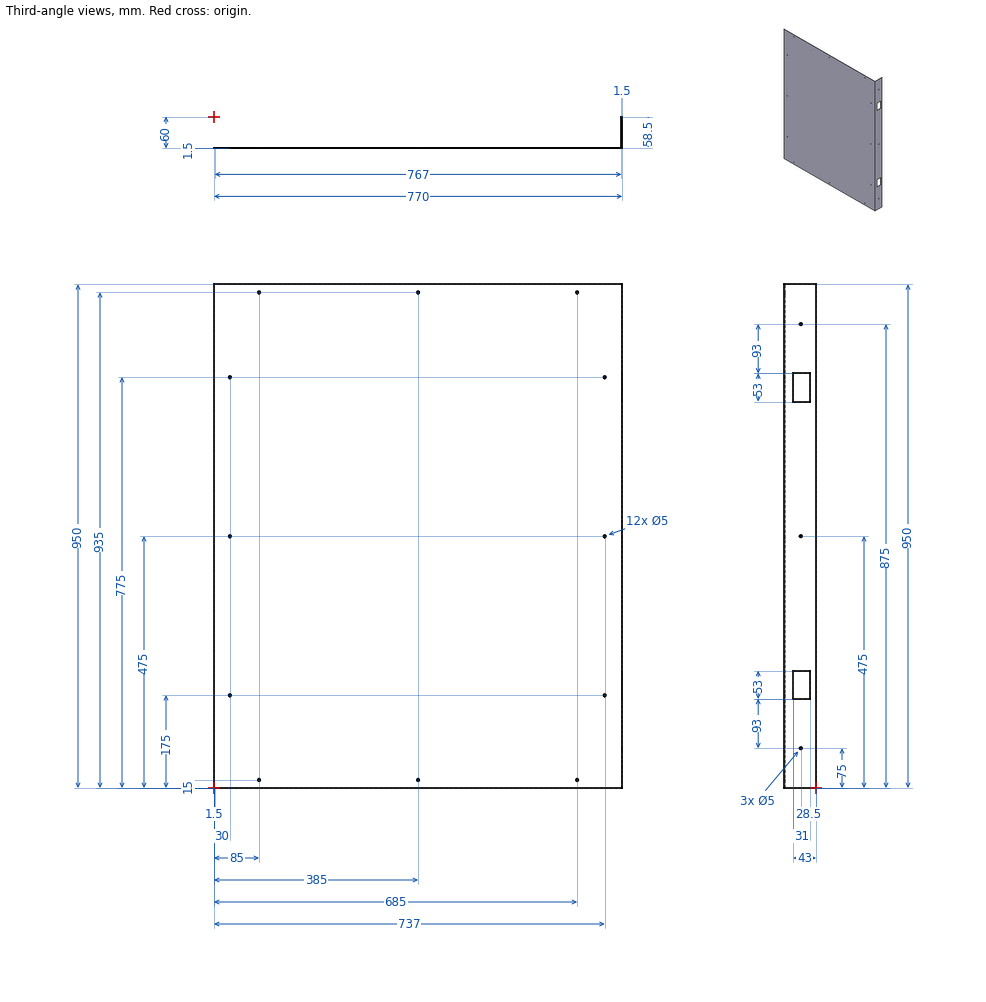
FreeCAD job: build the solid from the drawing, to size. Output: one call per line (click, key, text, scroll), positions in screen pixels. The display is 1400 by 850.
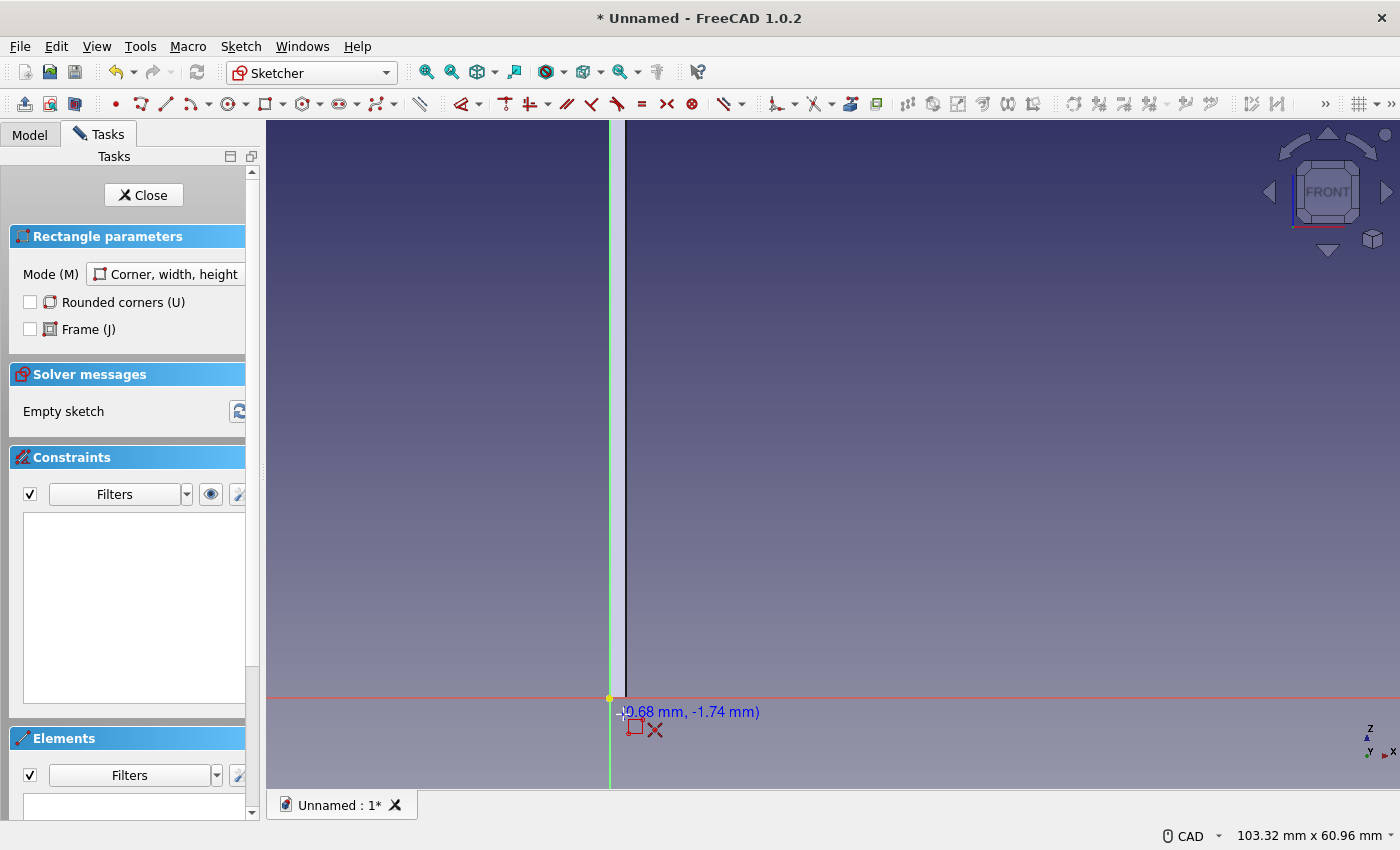
scroll(772, 715, down, 15)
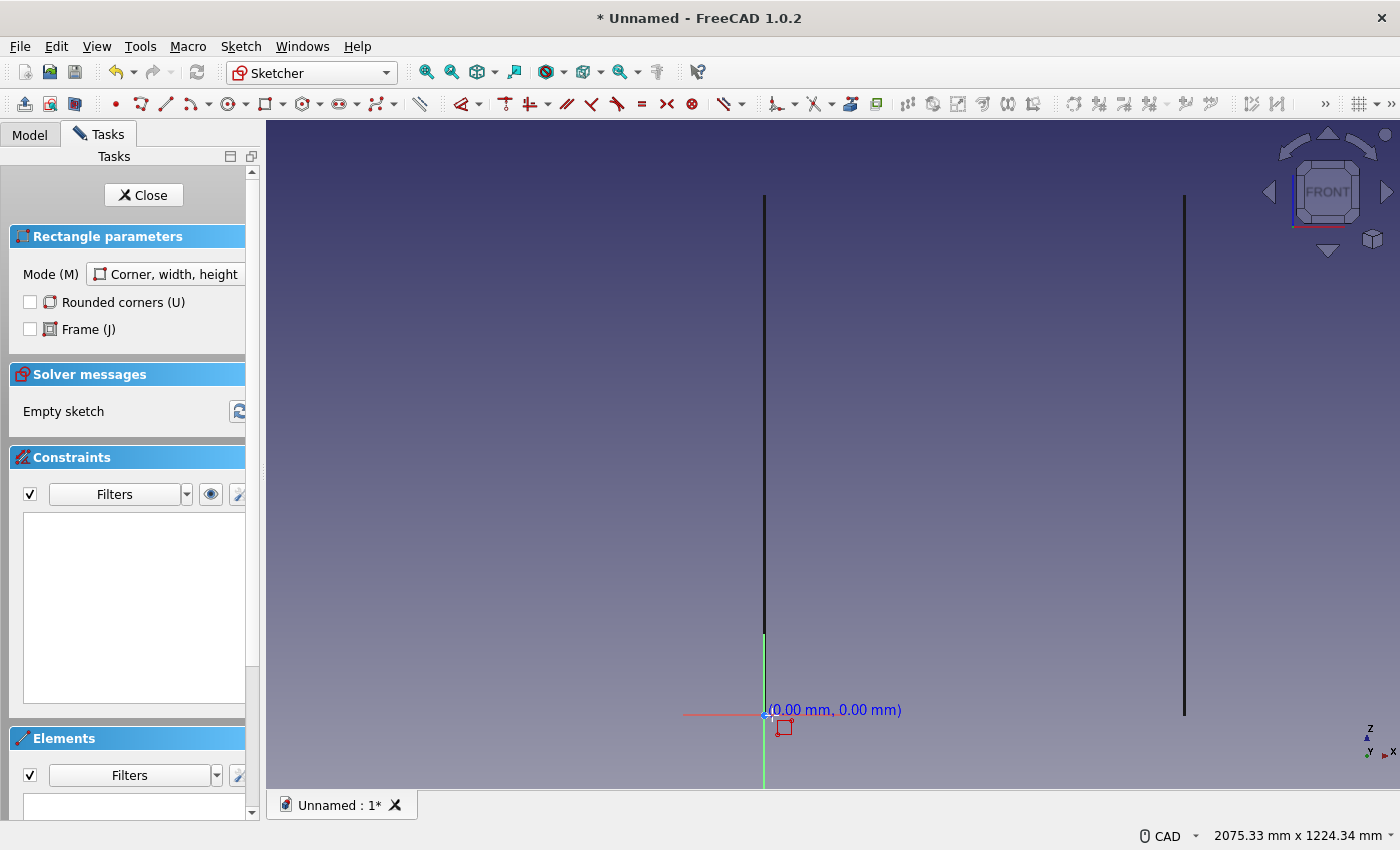
click(764, 715)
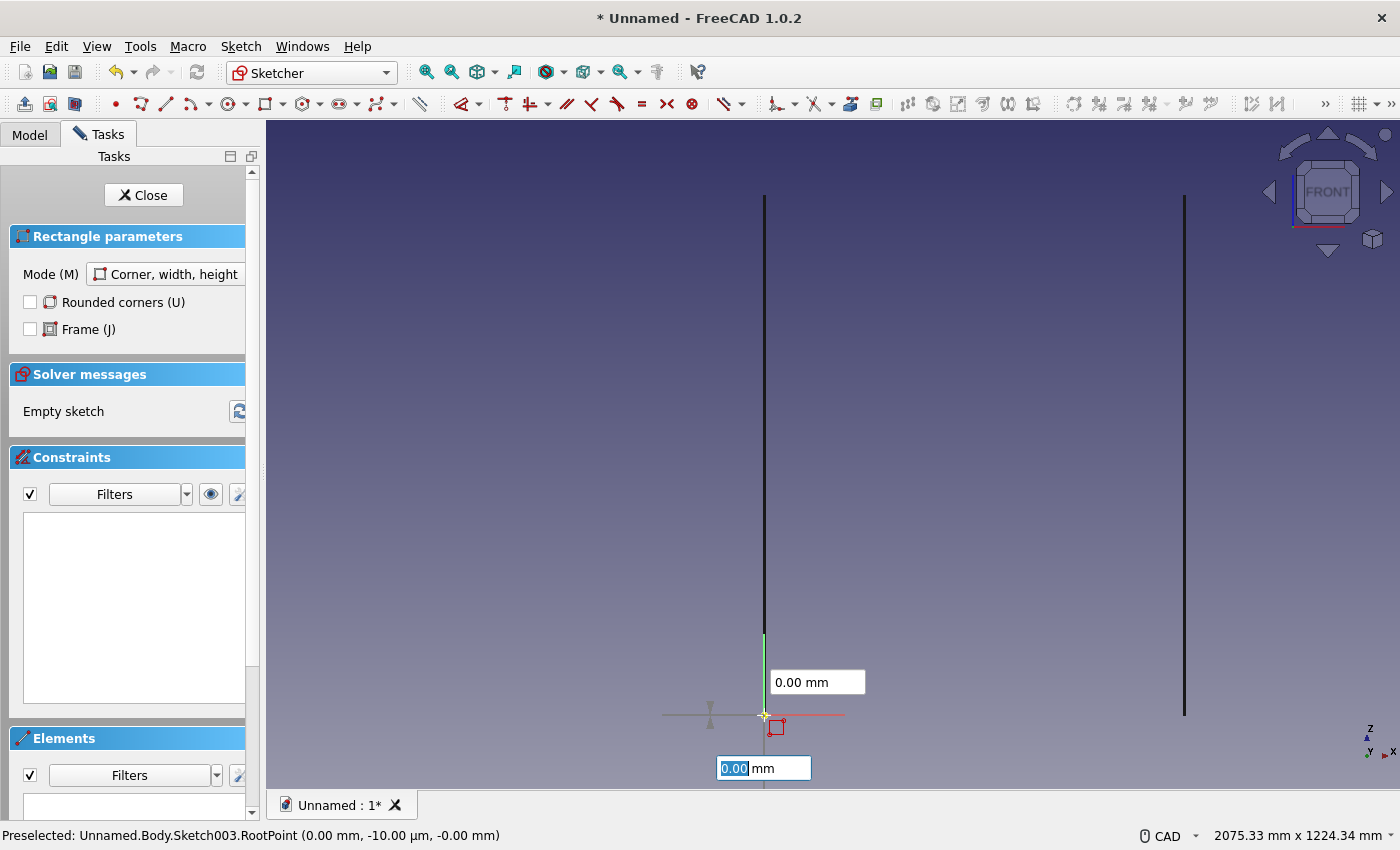
scroll(765, 196, up, 15)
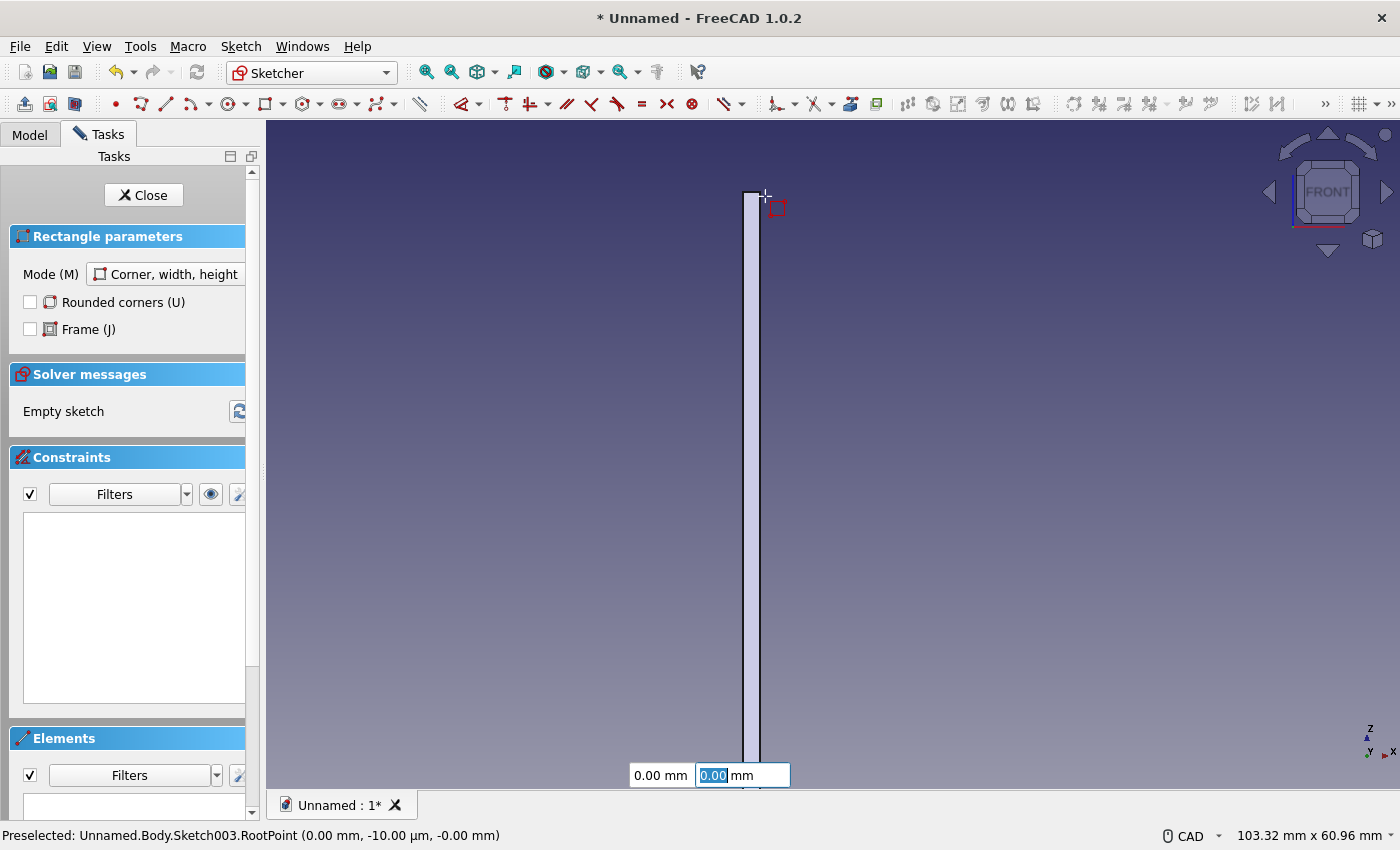
click(760, 192)
key(Escape)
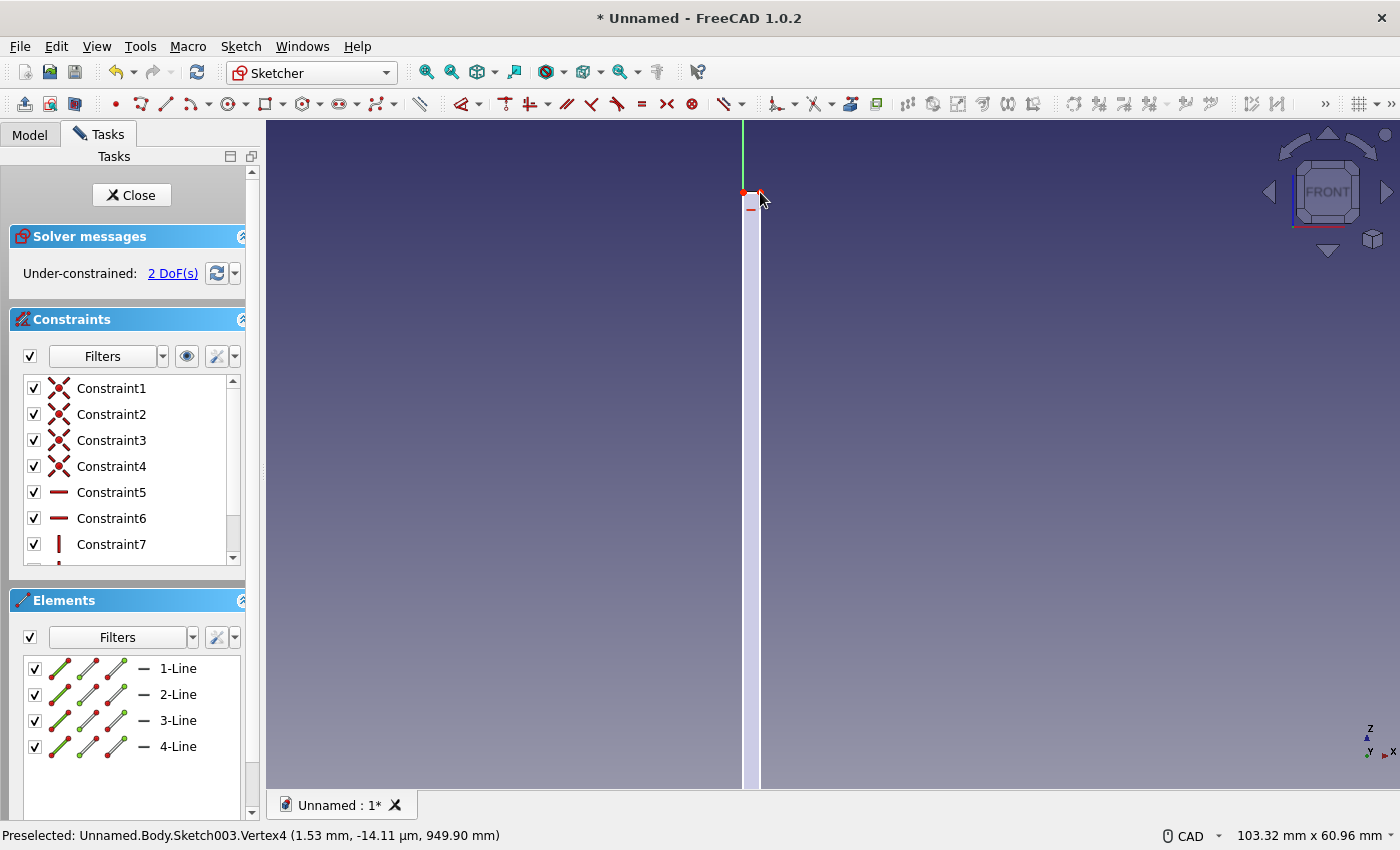
key(d)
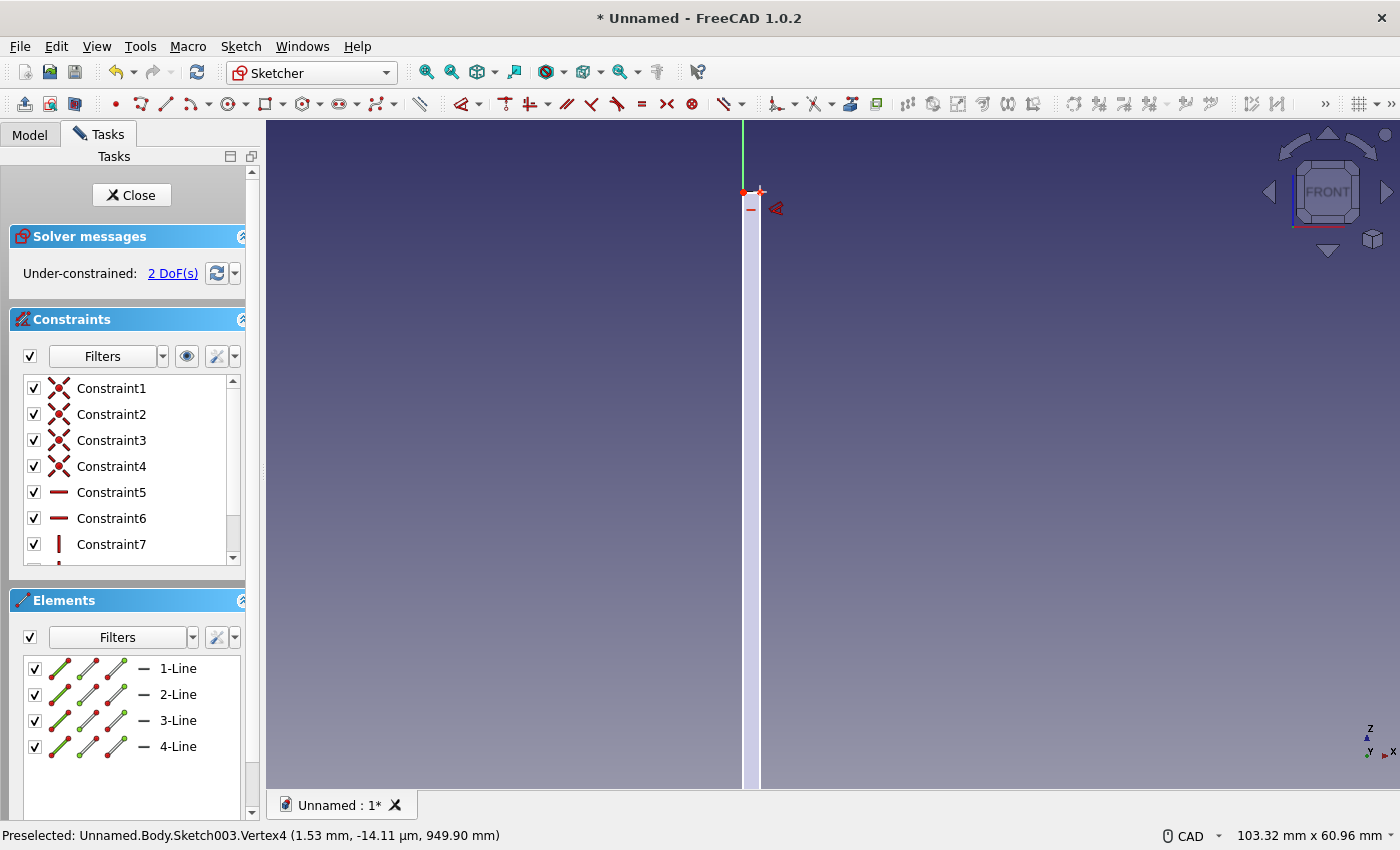
scroll(765, 195, down, 15)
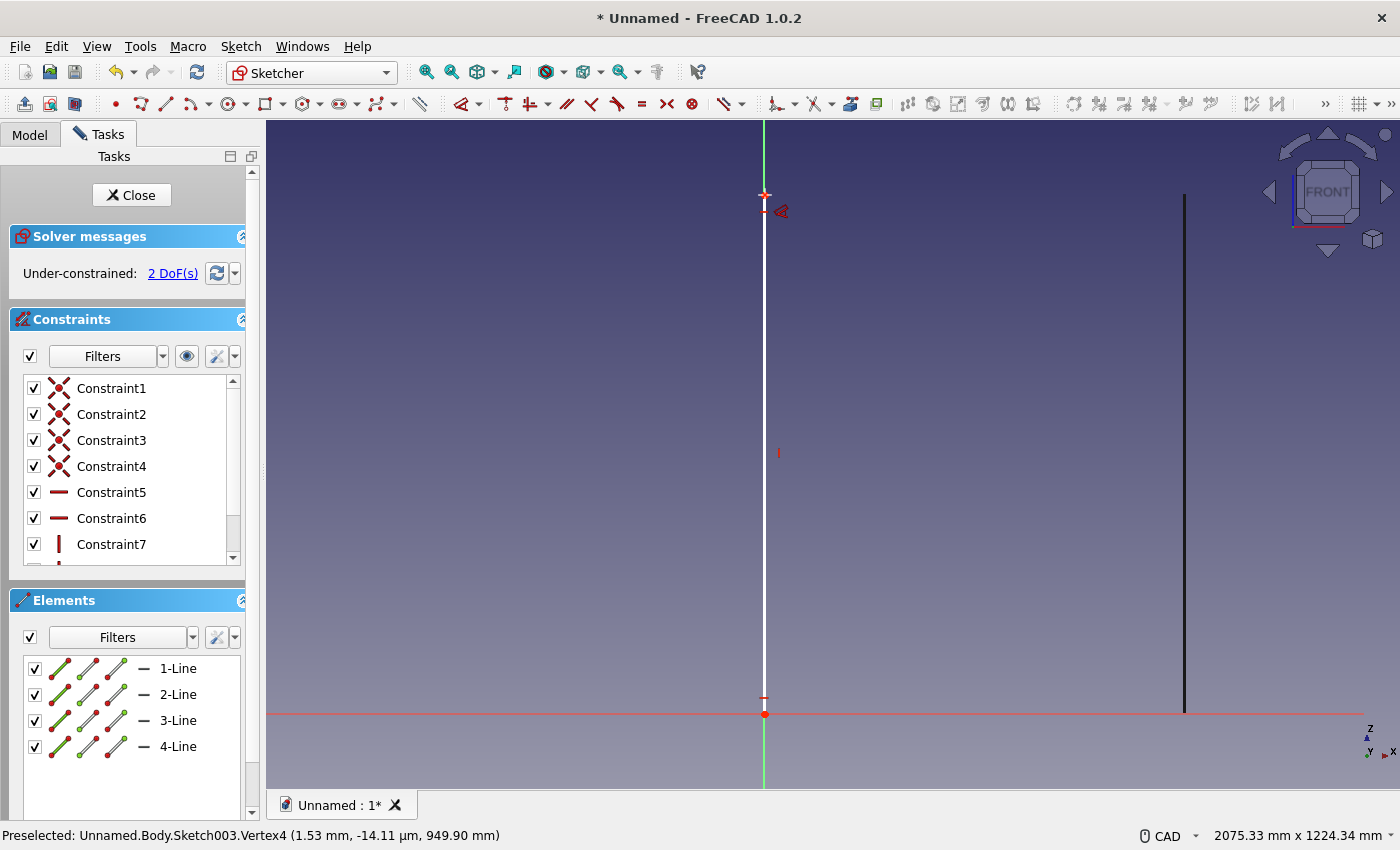
scroll(765, 714, up, 20)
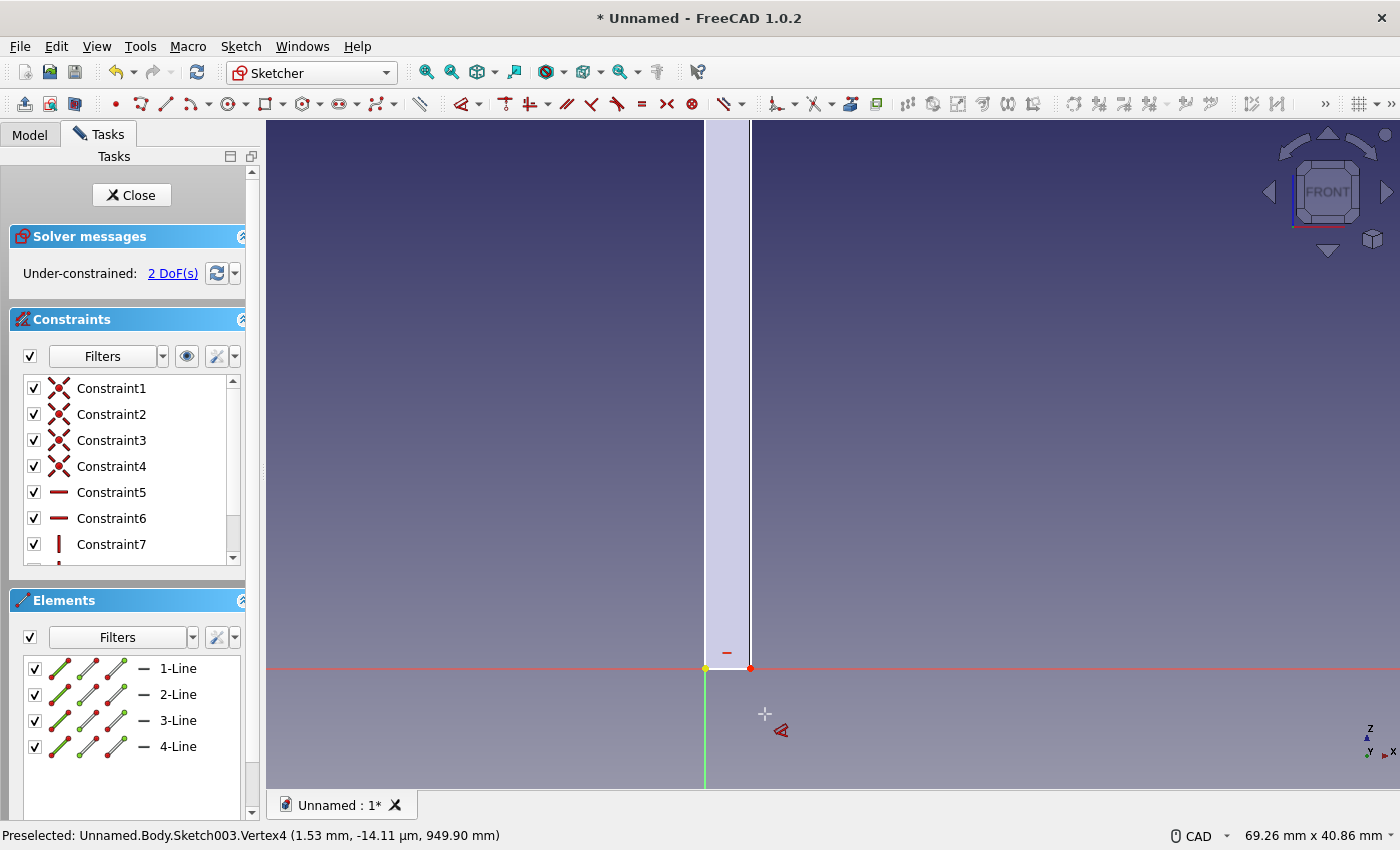
click(728, 669)
click(728, 703)